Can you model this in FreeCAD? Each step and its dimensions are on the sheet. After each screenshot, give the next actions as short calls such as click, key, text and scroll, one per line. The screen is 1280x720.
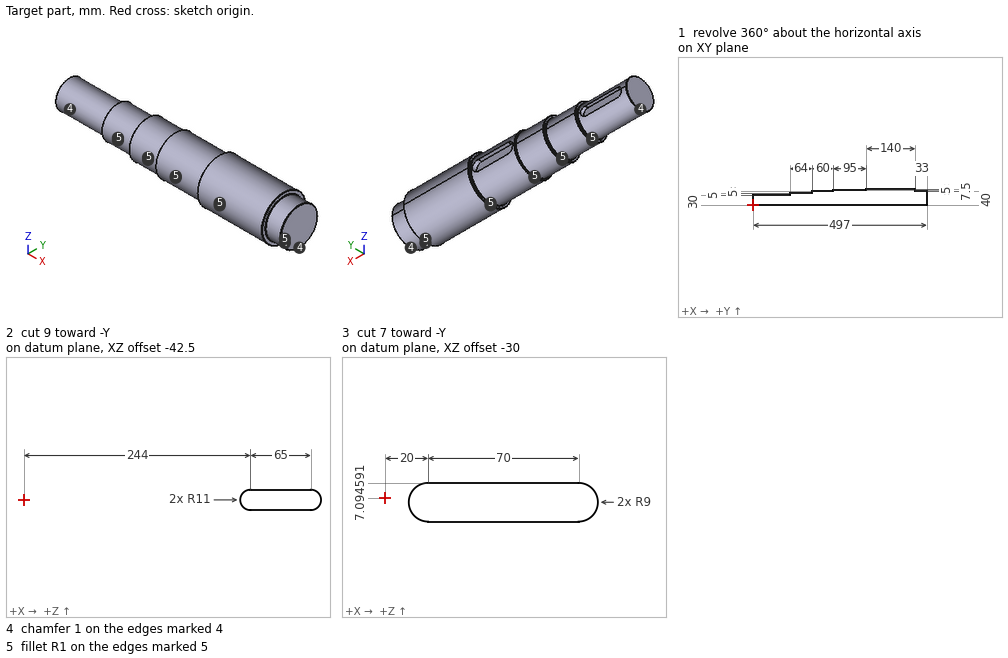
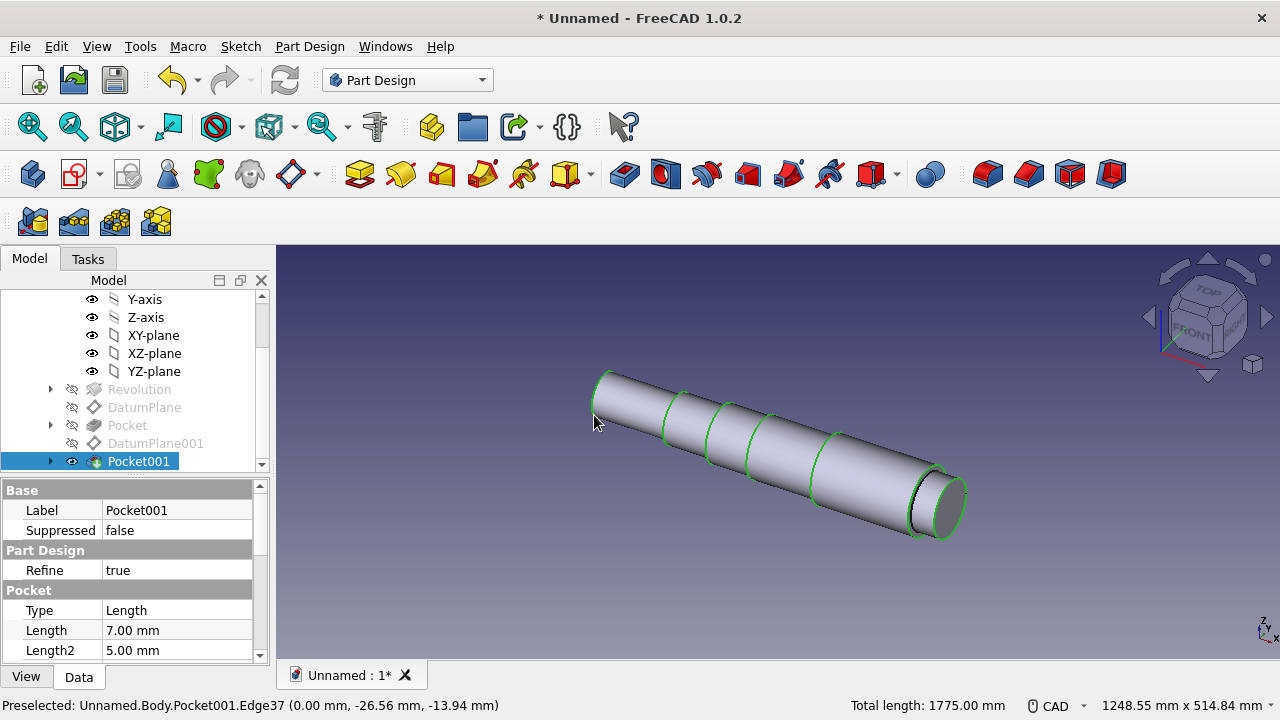
click(1029, 174)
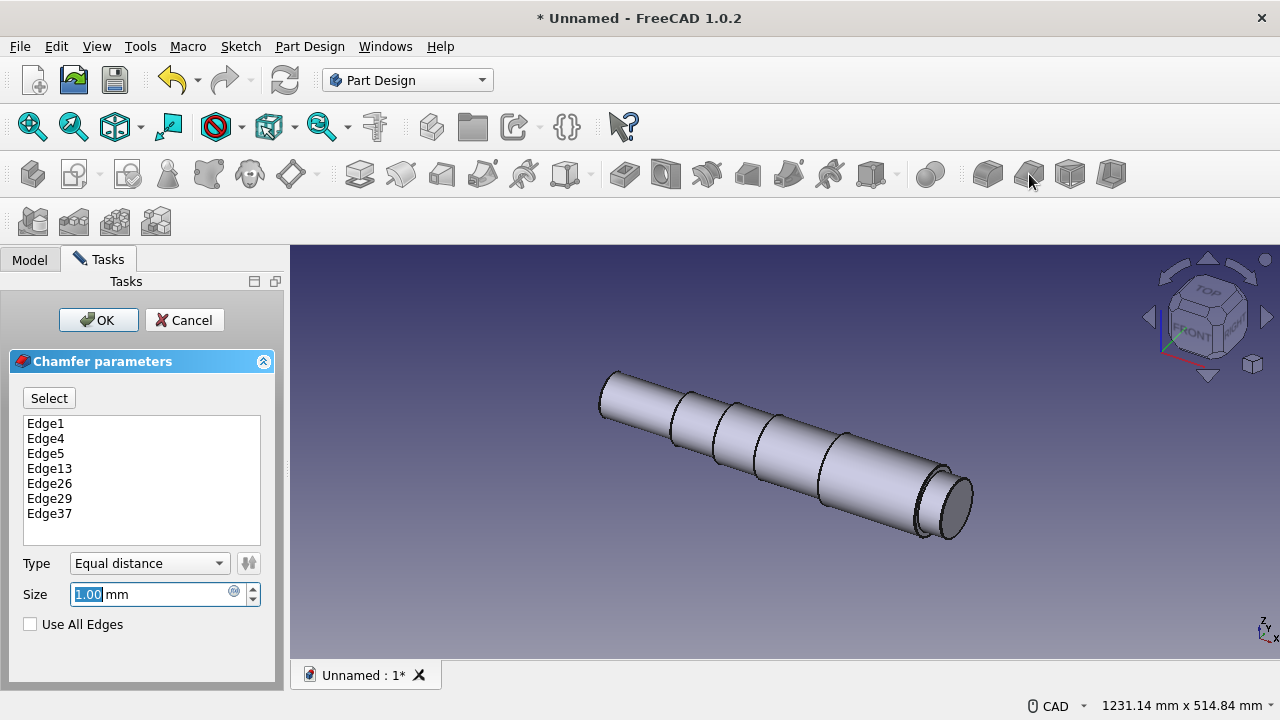
text(1)
key(Tab)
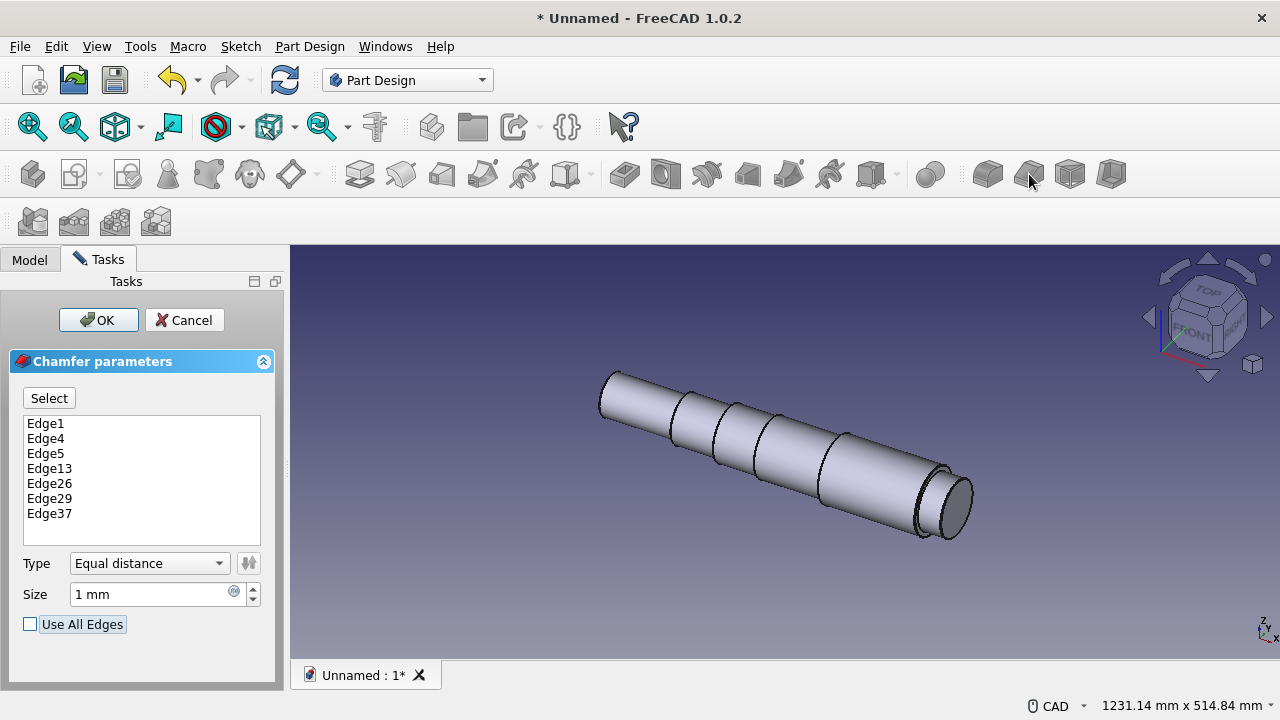
click(99, 320)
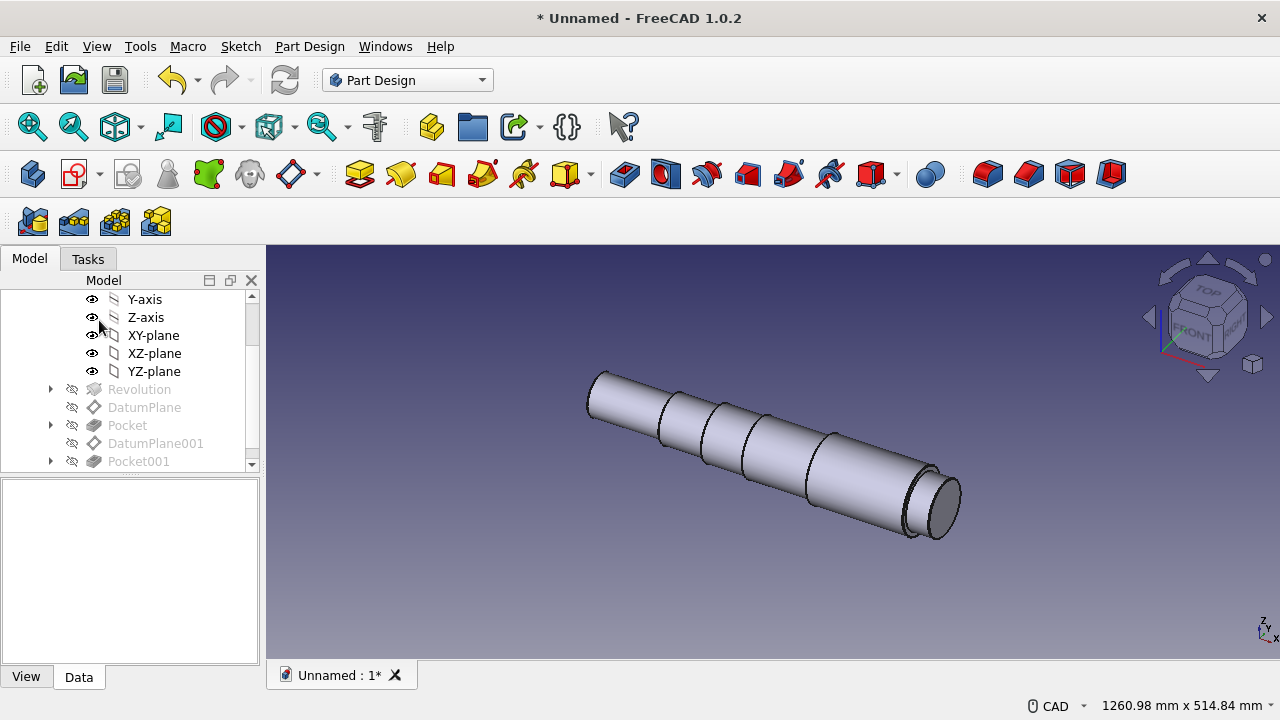
key(0)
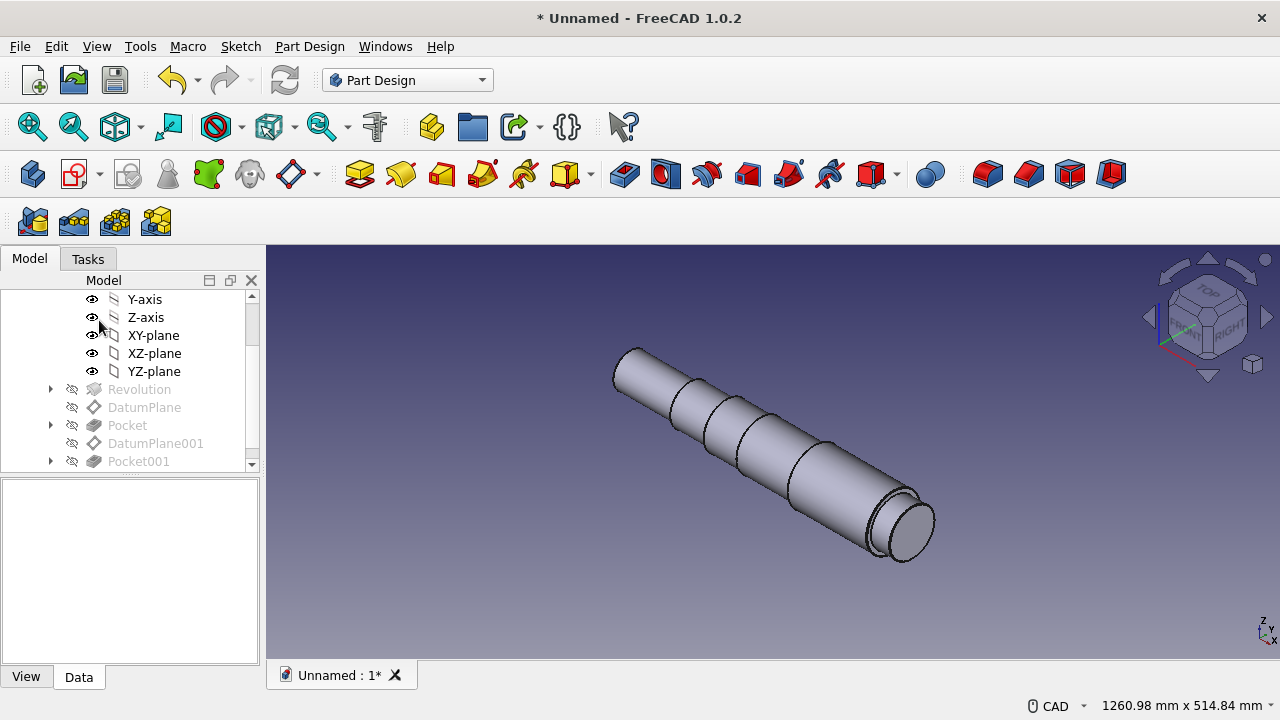
key(2)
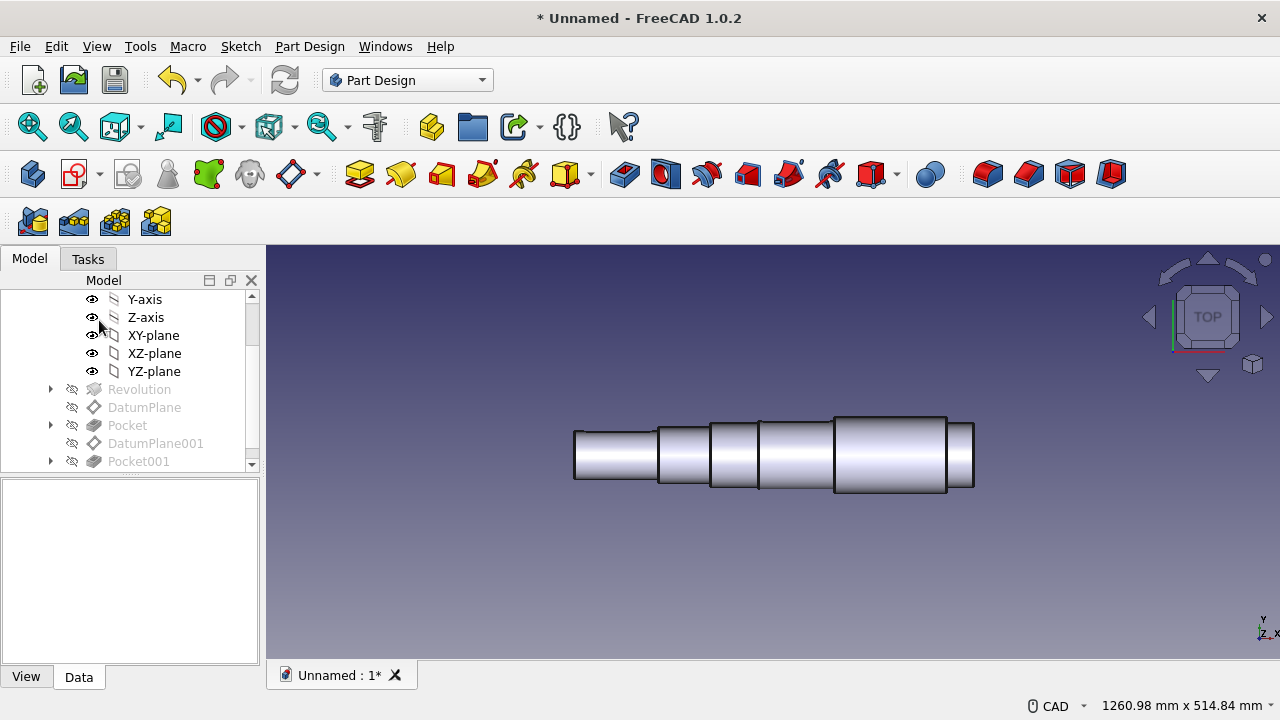
click(33, 128)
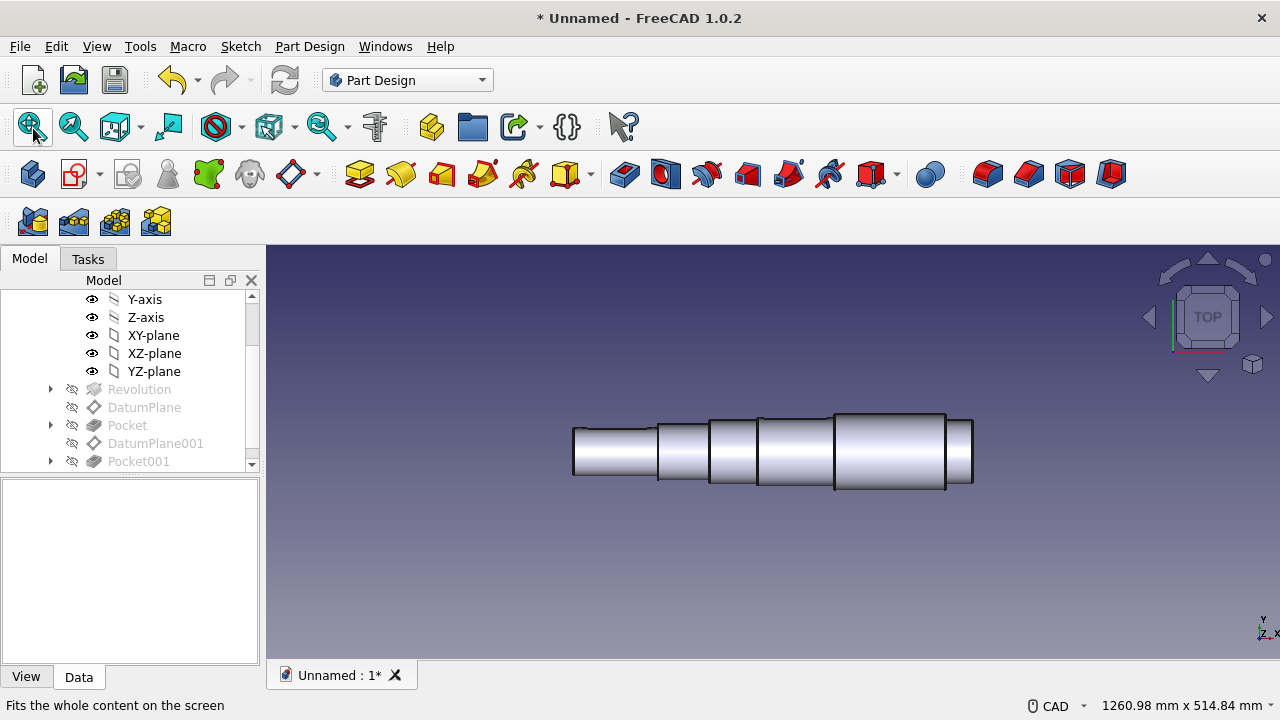
key(1)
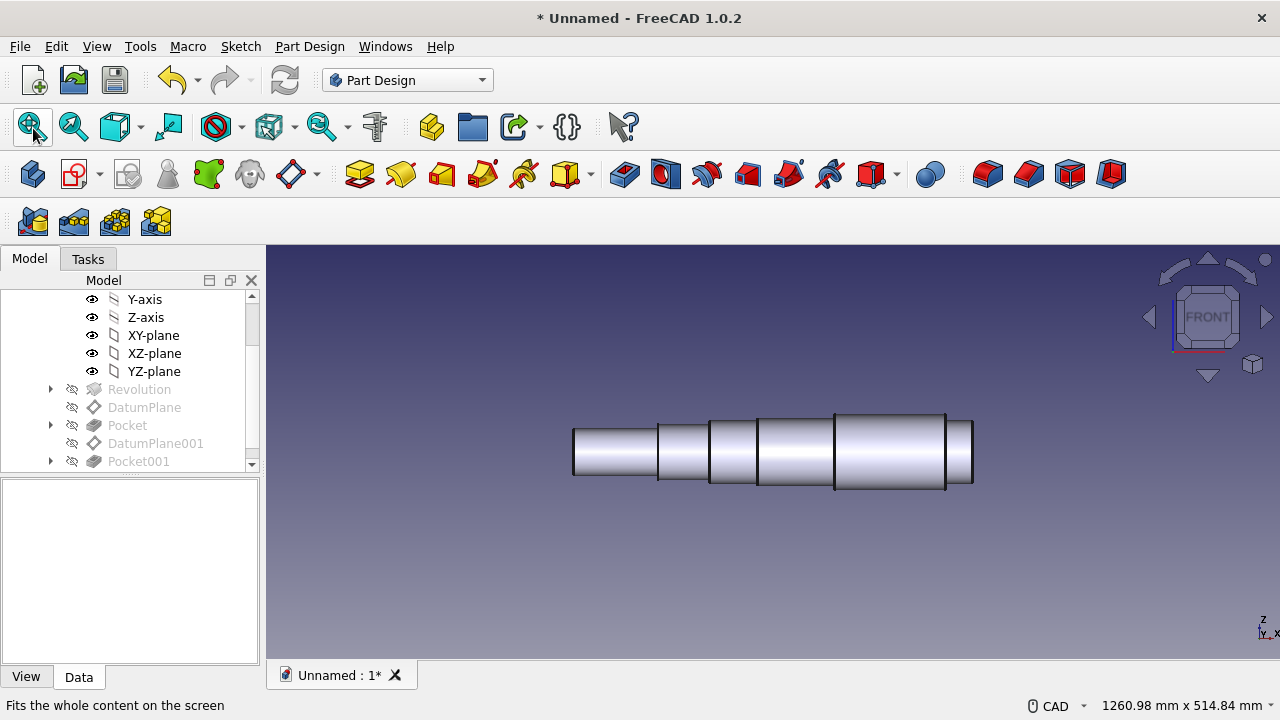
click(33, 128)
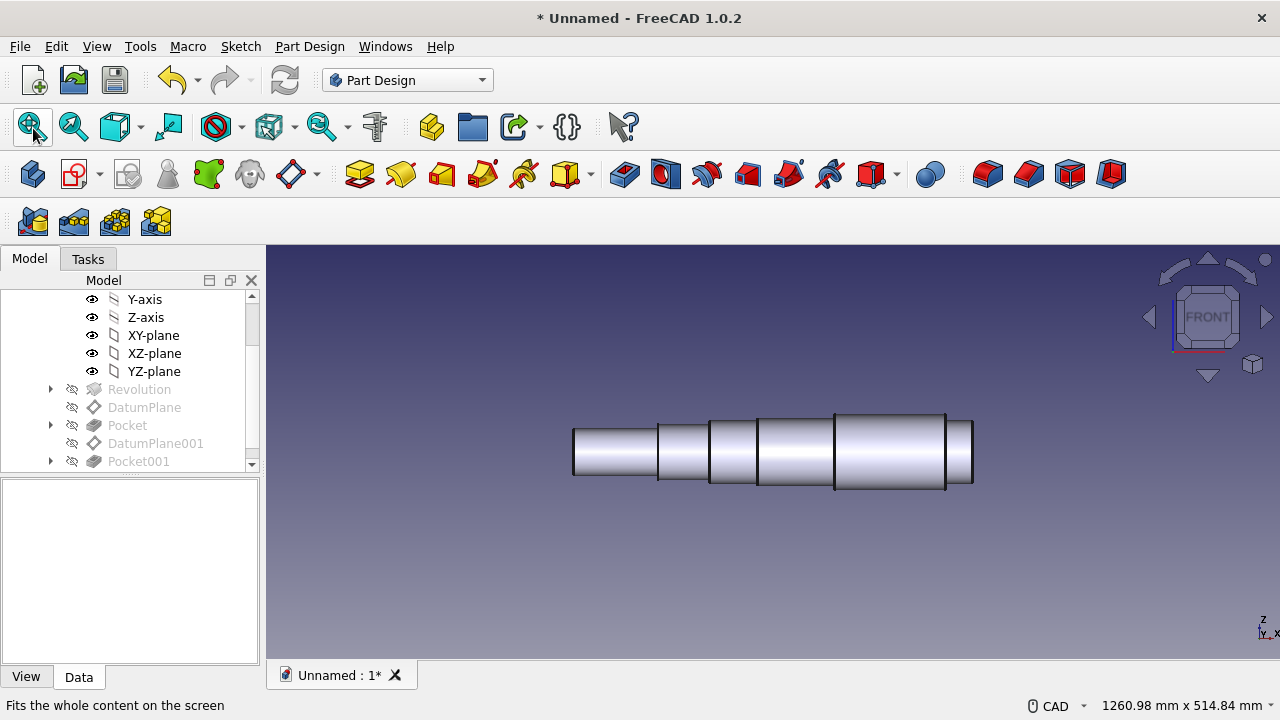
key(3)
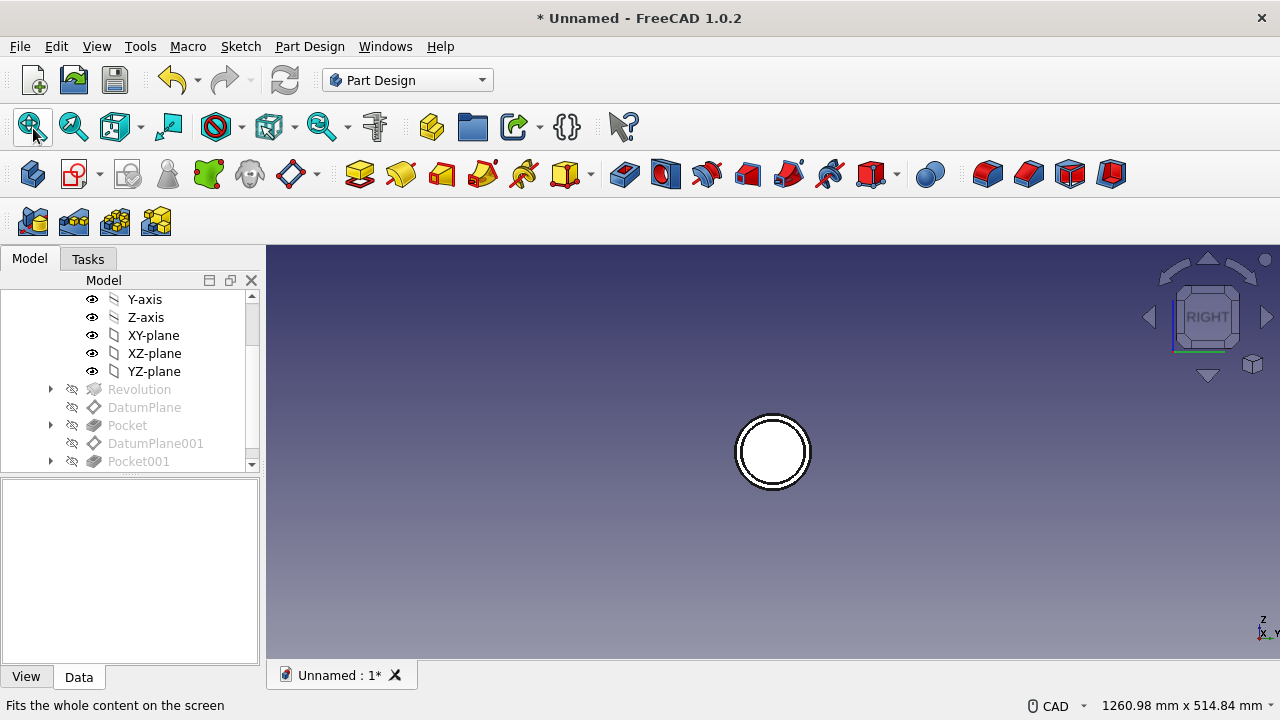
click(33, 128)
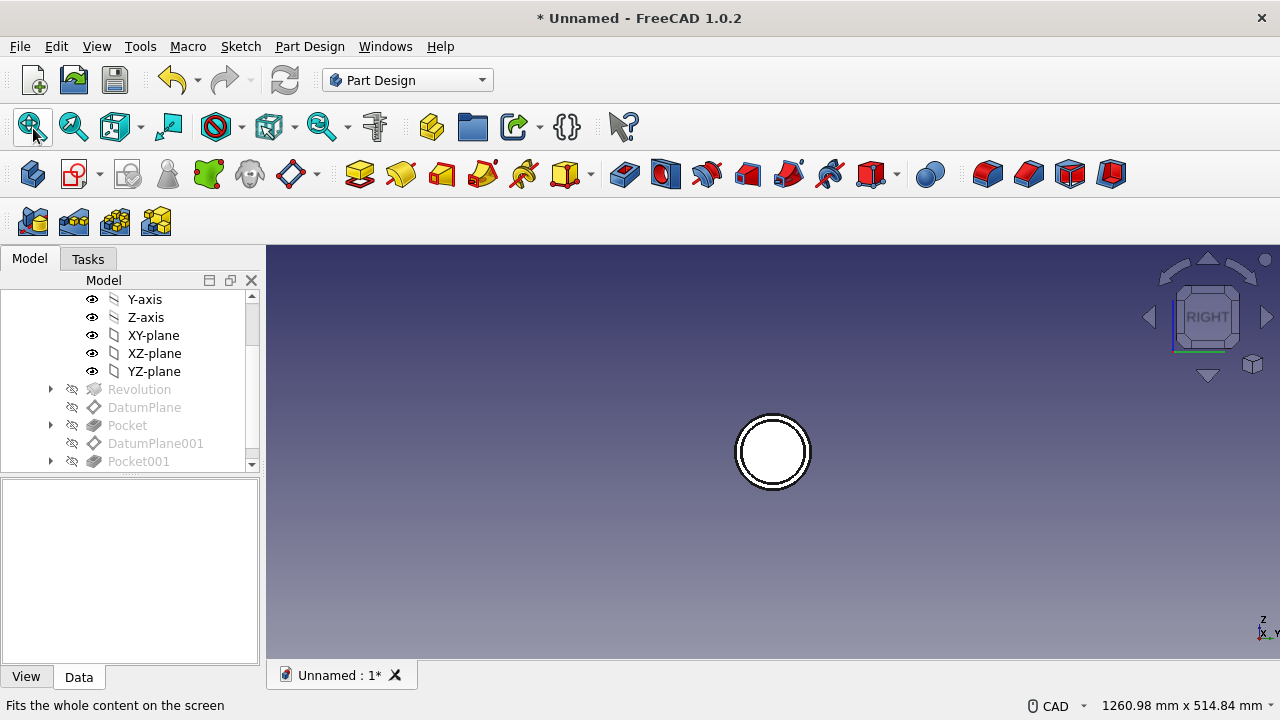
key(5)